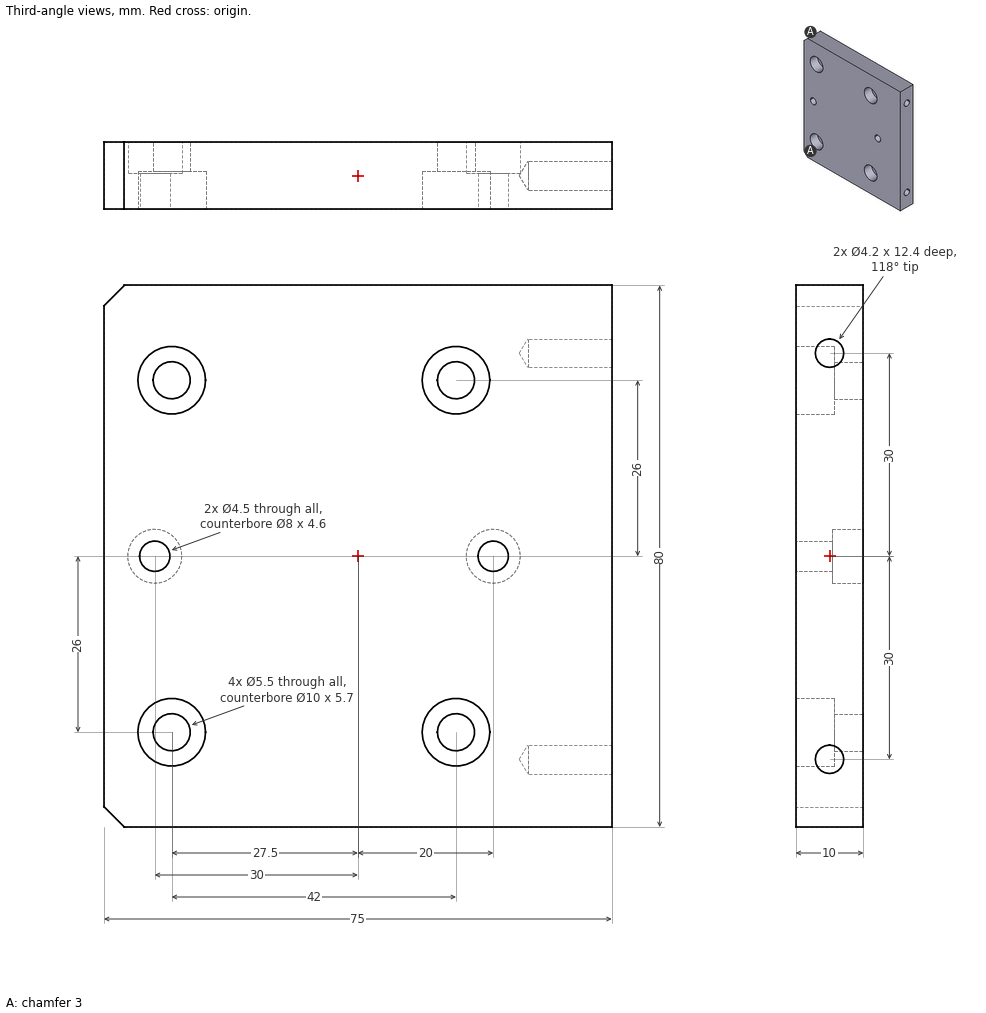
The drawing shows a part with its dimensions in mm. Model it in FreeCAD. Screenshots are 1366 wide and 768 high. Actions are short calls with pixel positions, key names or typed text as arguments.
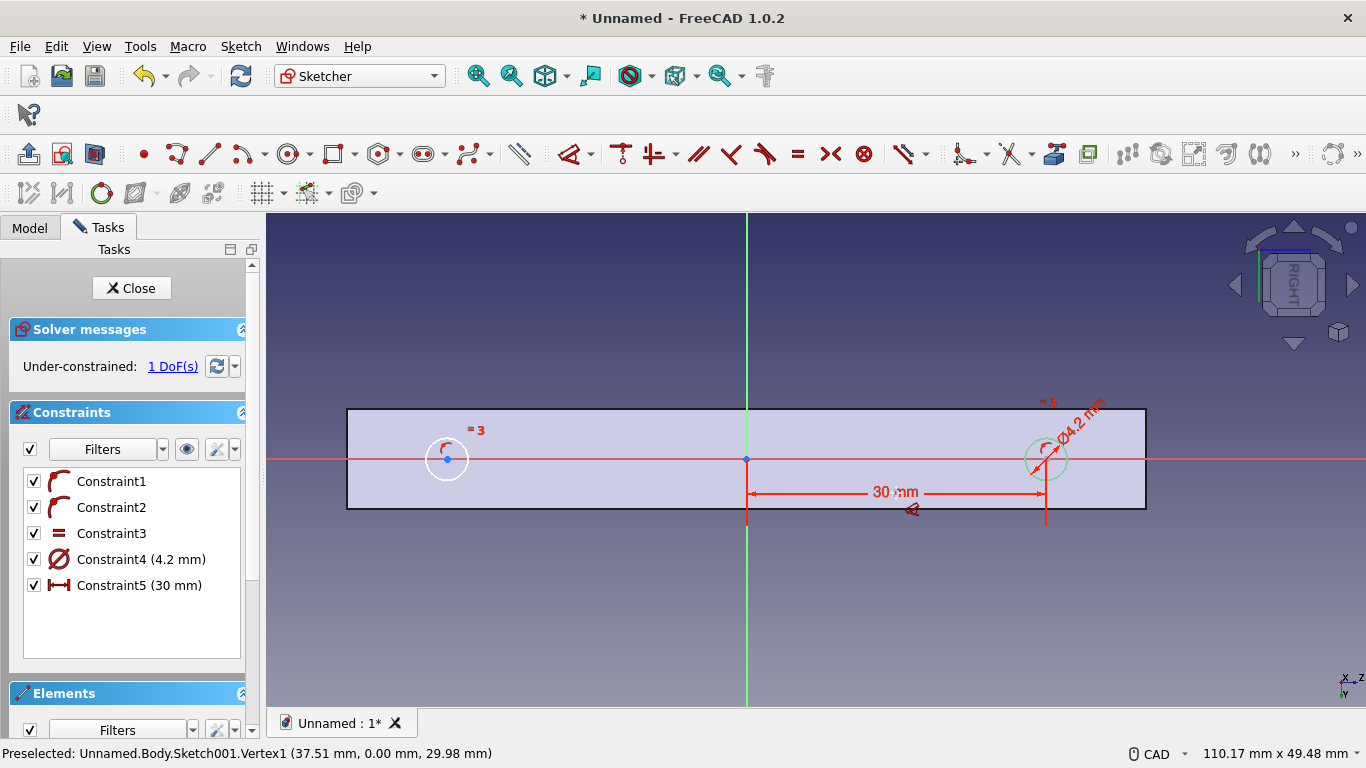
click(447, 459)
click(597, 493)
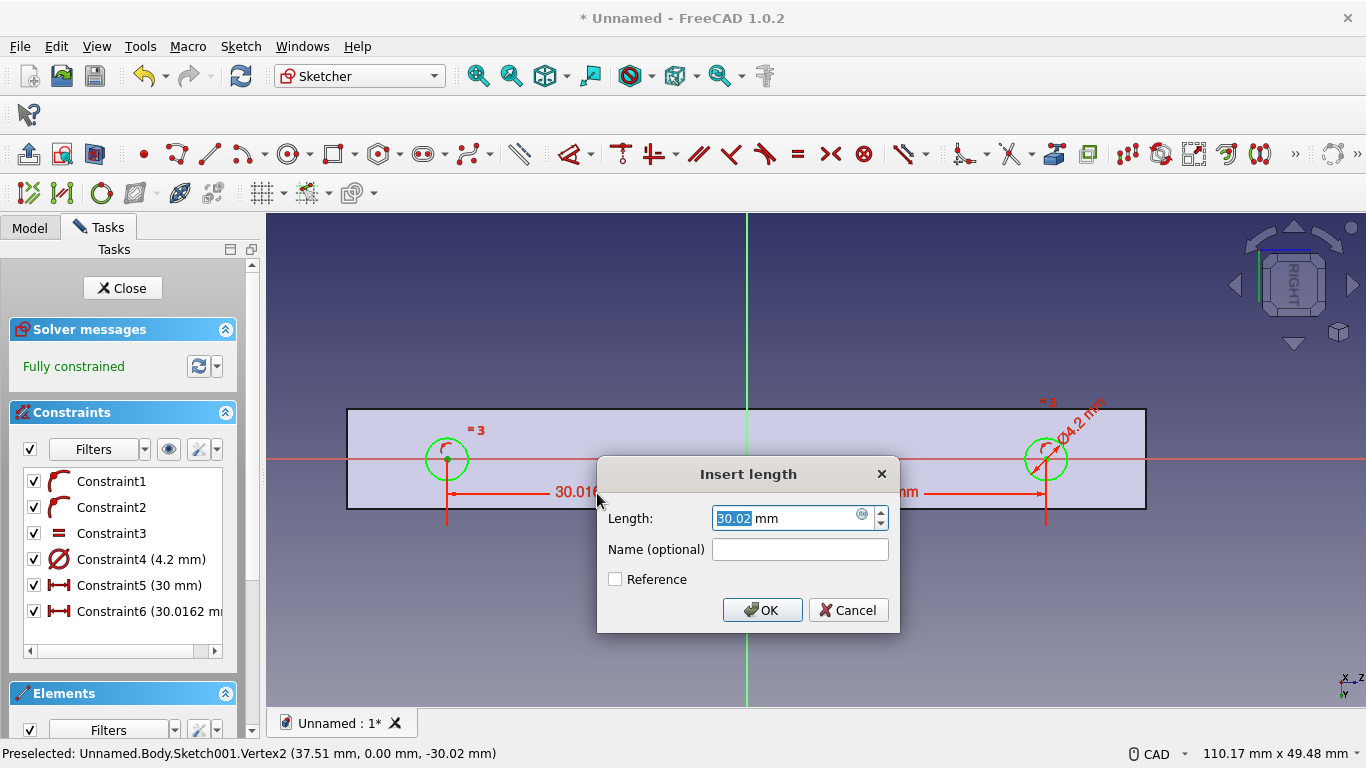
text(30)
key(Return)
key(Escape)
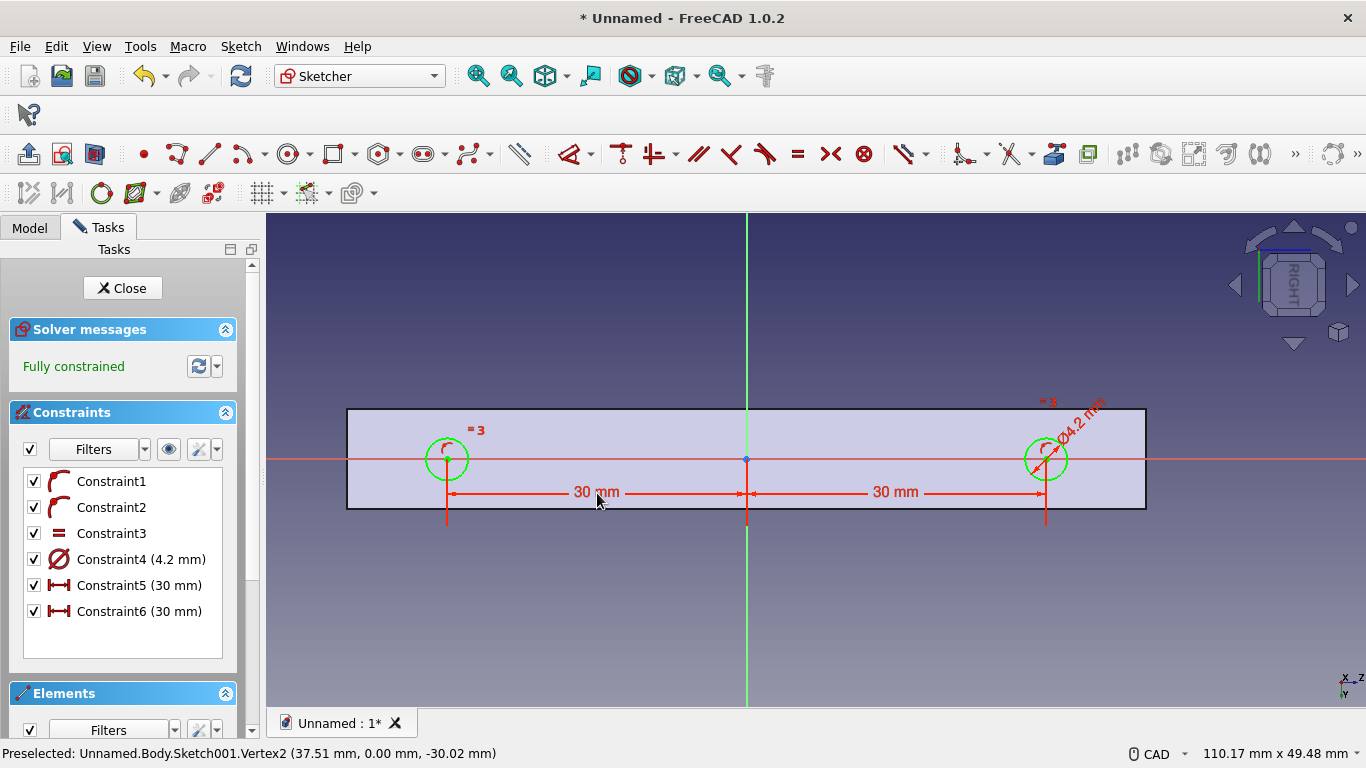
click(123, 288)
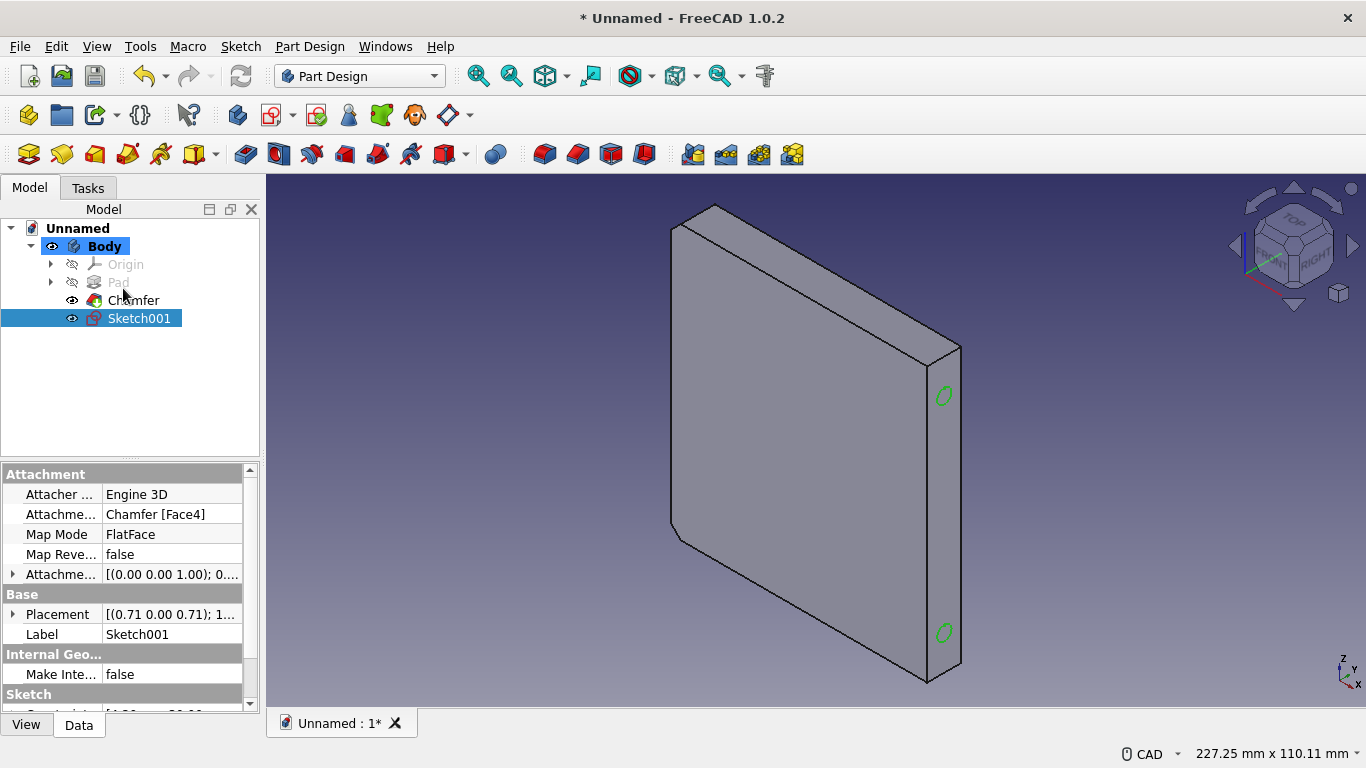
click(279, 154)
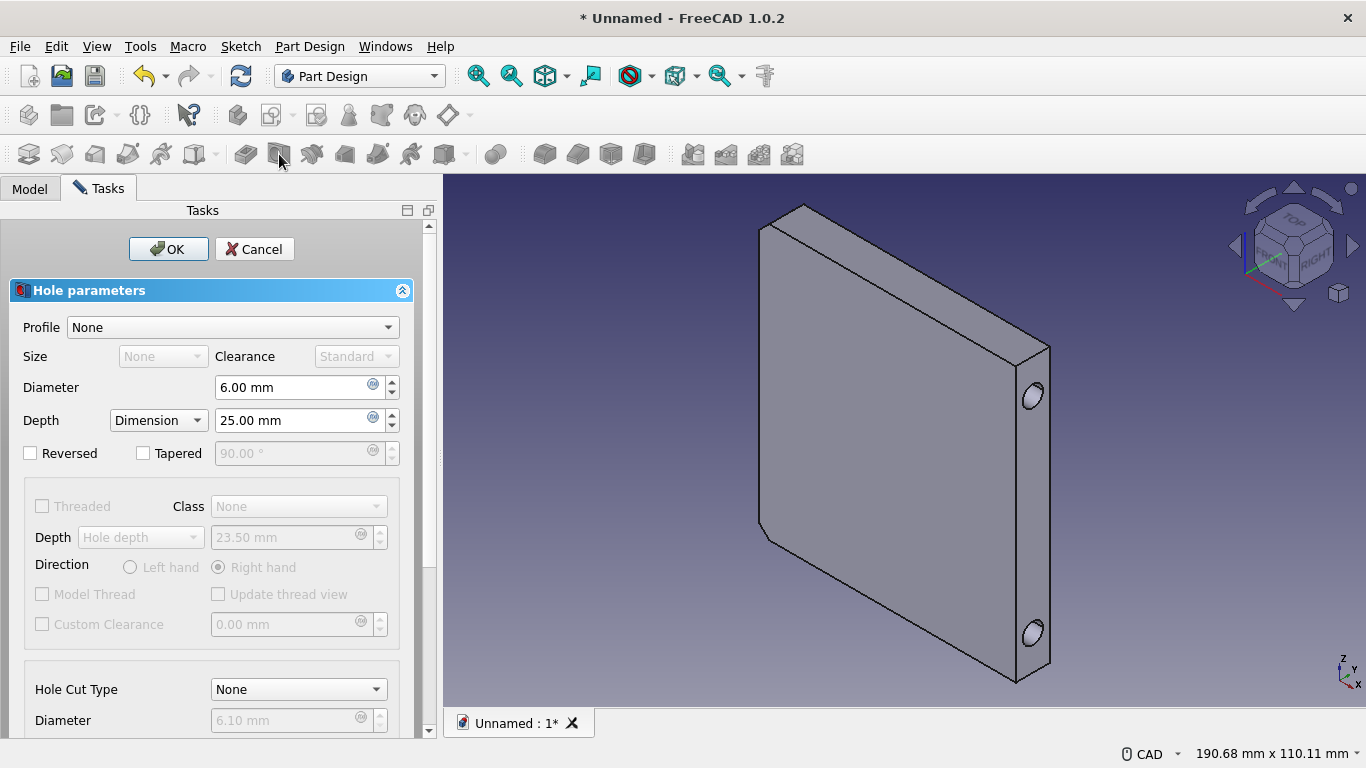
triple_click(300, 388)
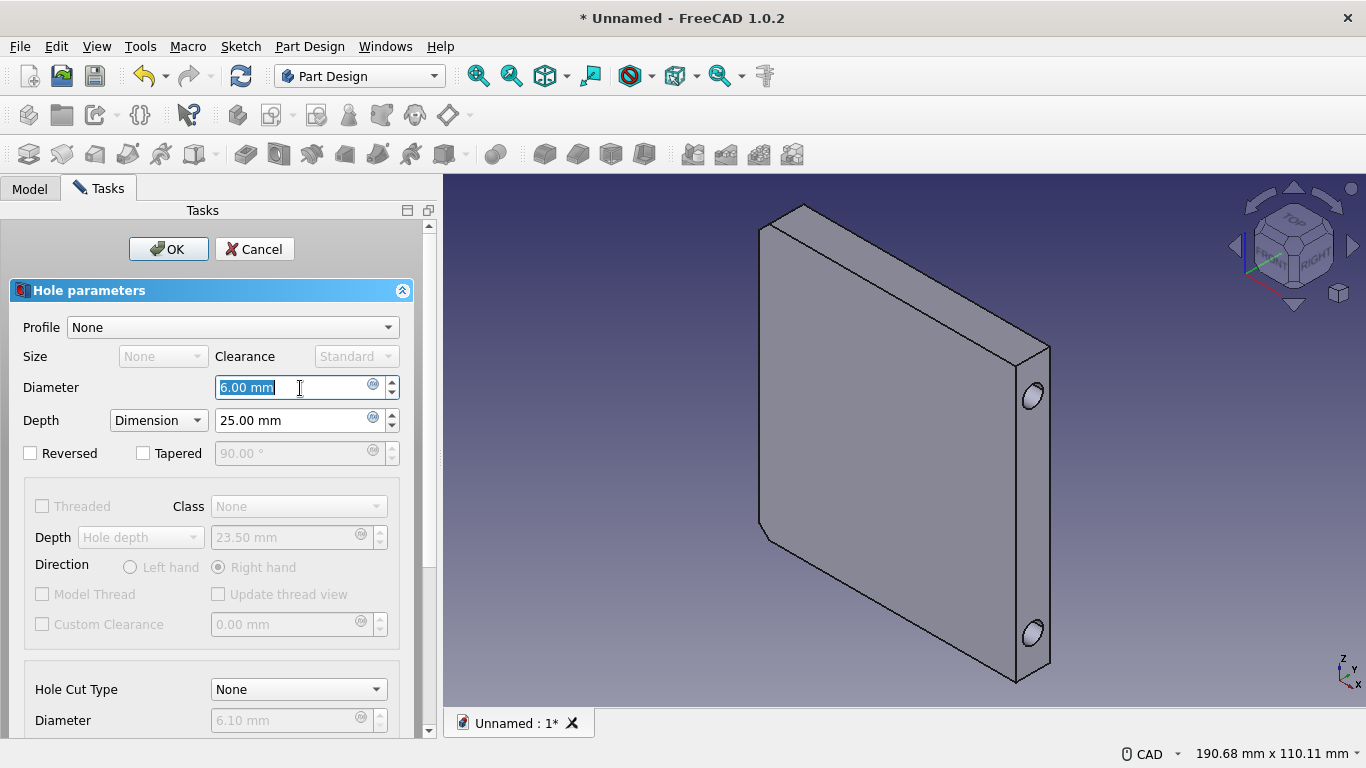
text(4.2)
key(Tab)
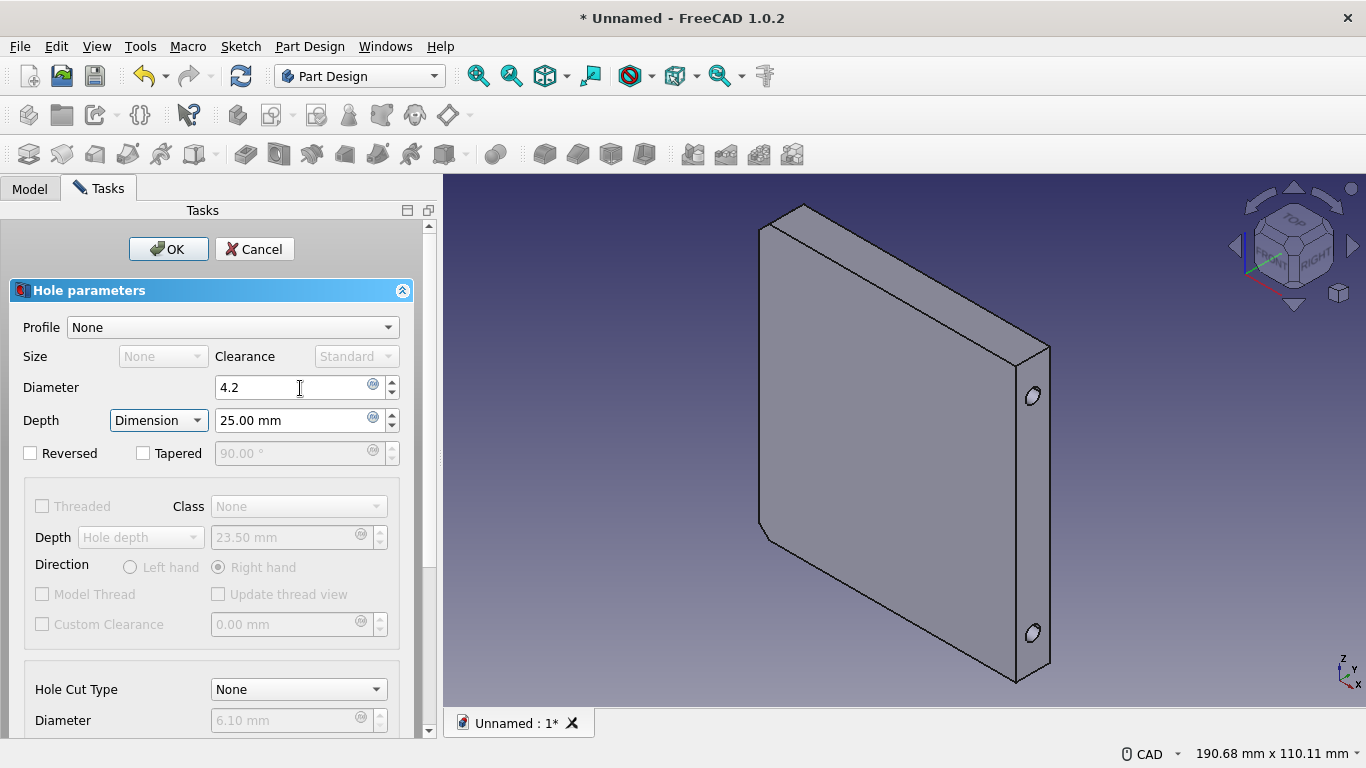
triple_click(300, 420)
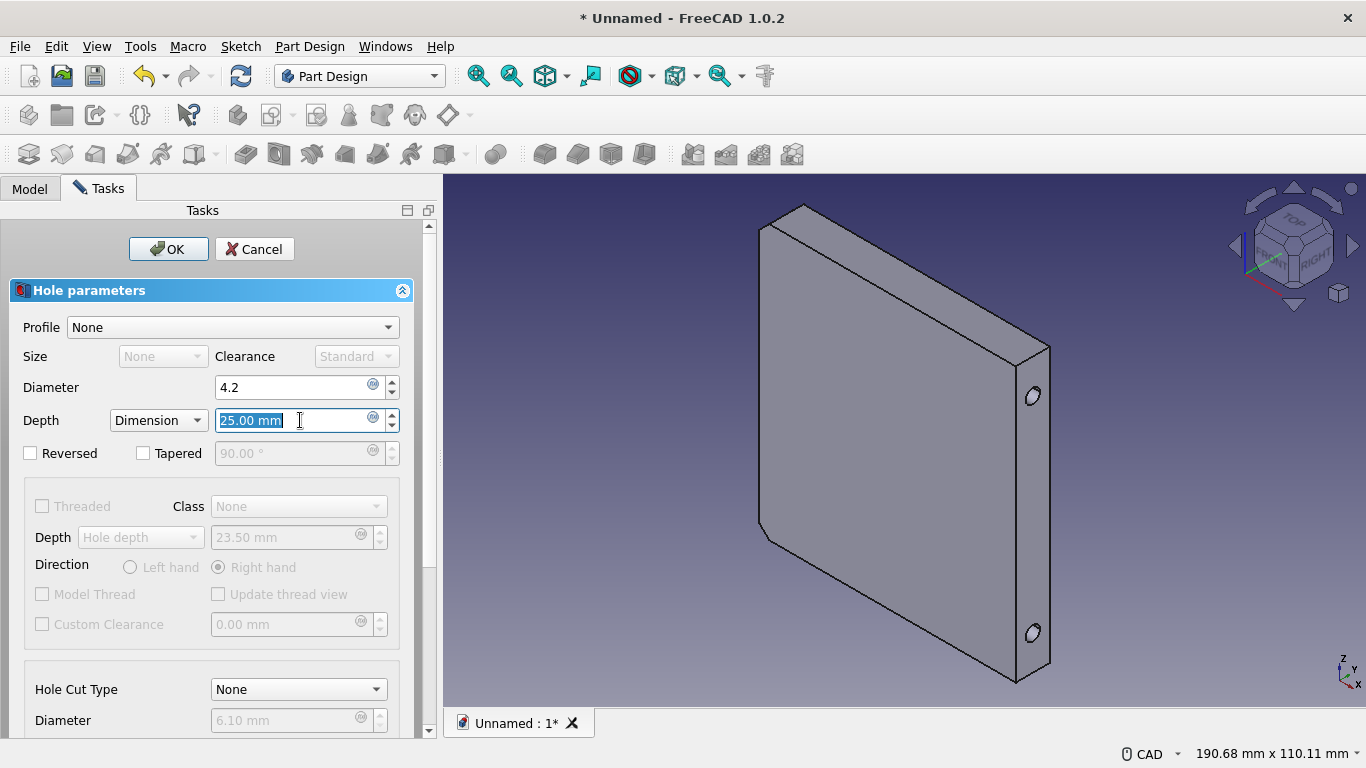
text(12.4)
key(Tab)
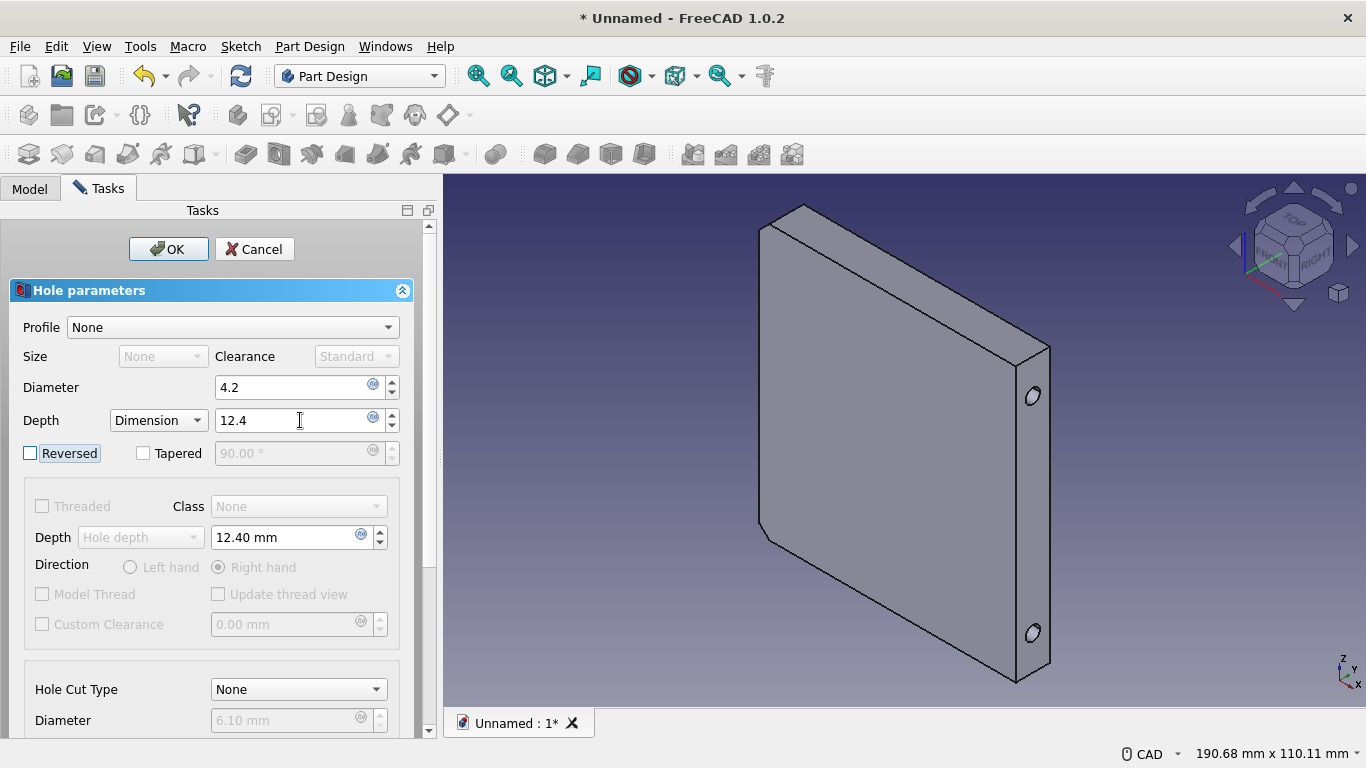
click(169, 249)